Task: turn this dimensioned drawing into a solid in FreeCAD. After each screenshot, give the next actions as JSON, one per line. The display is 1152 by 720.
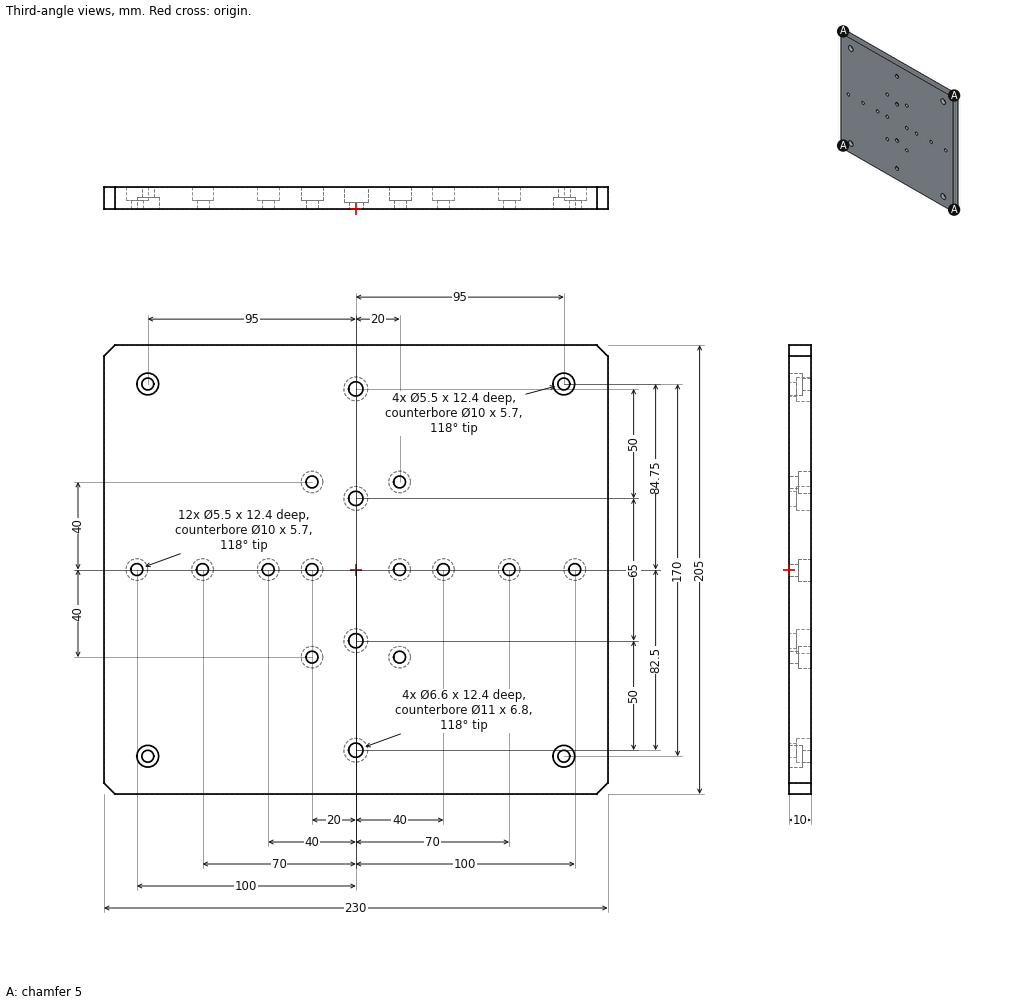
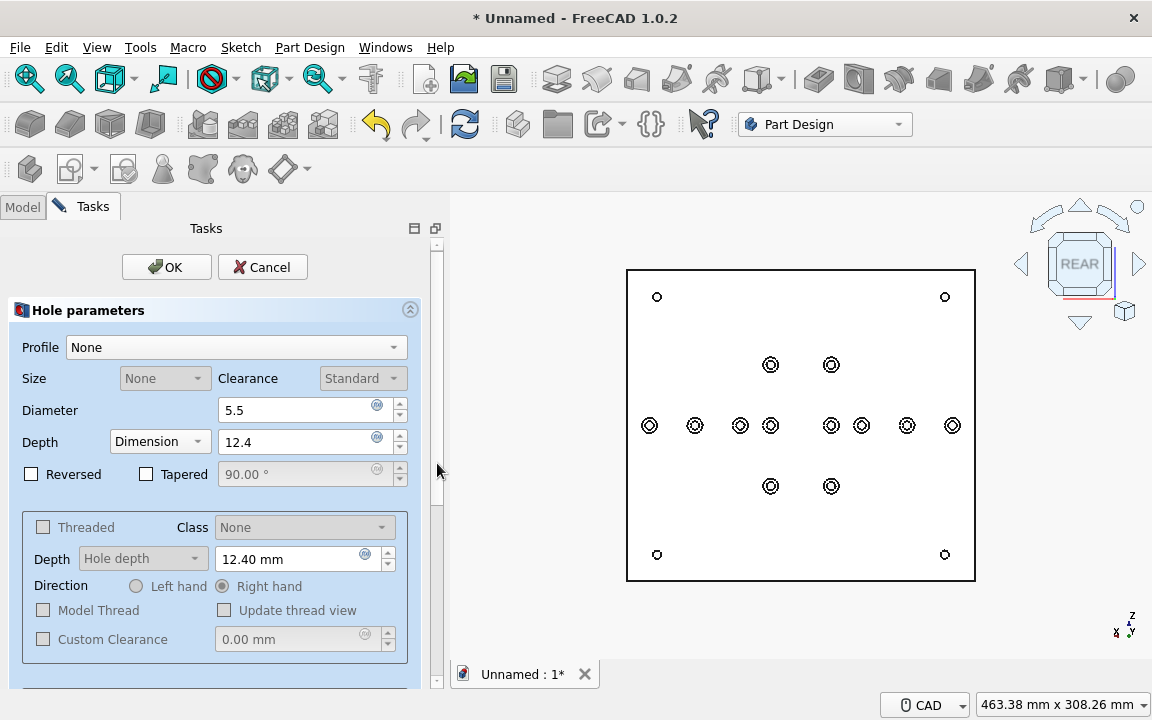
{"action": "left_click", "coordinate": [167, 267]}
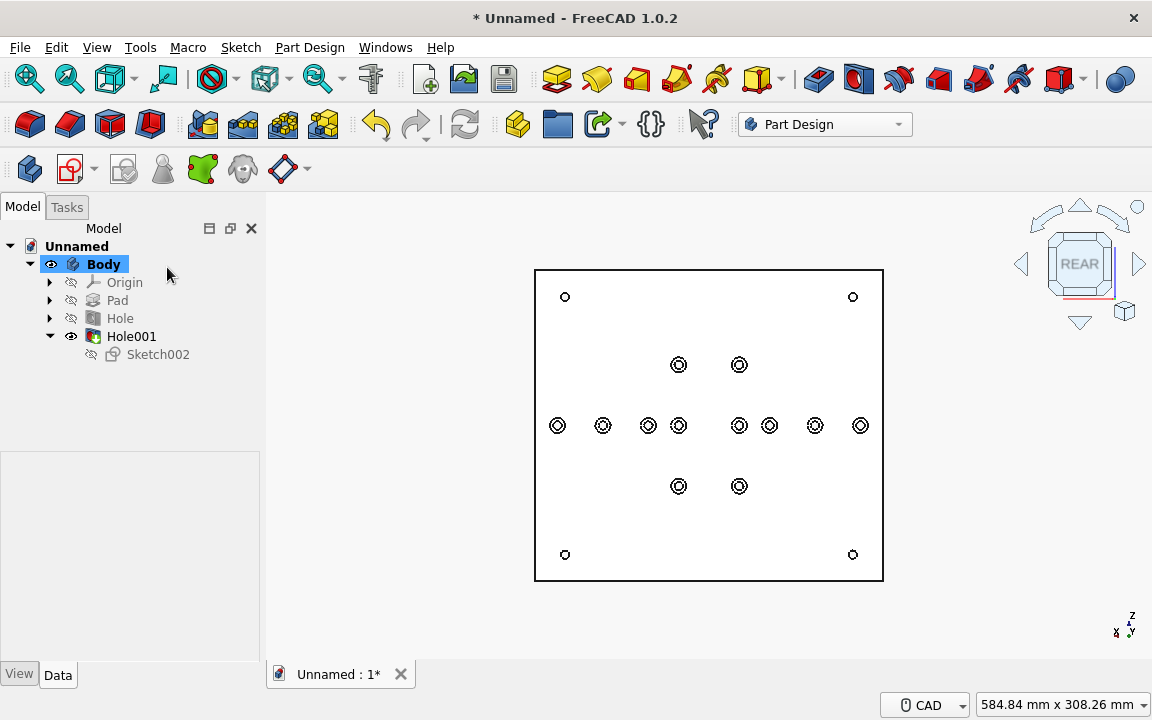
{"action": "scroll", "coordinate": [535, 269], "scroll_direction": "up", "scroll_amount": 5}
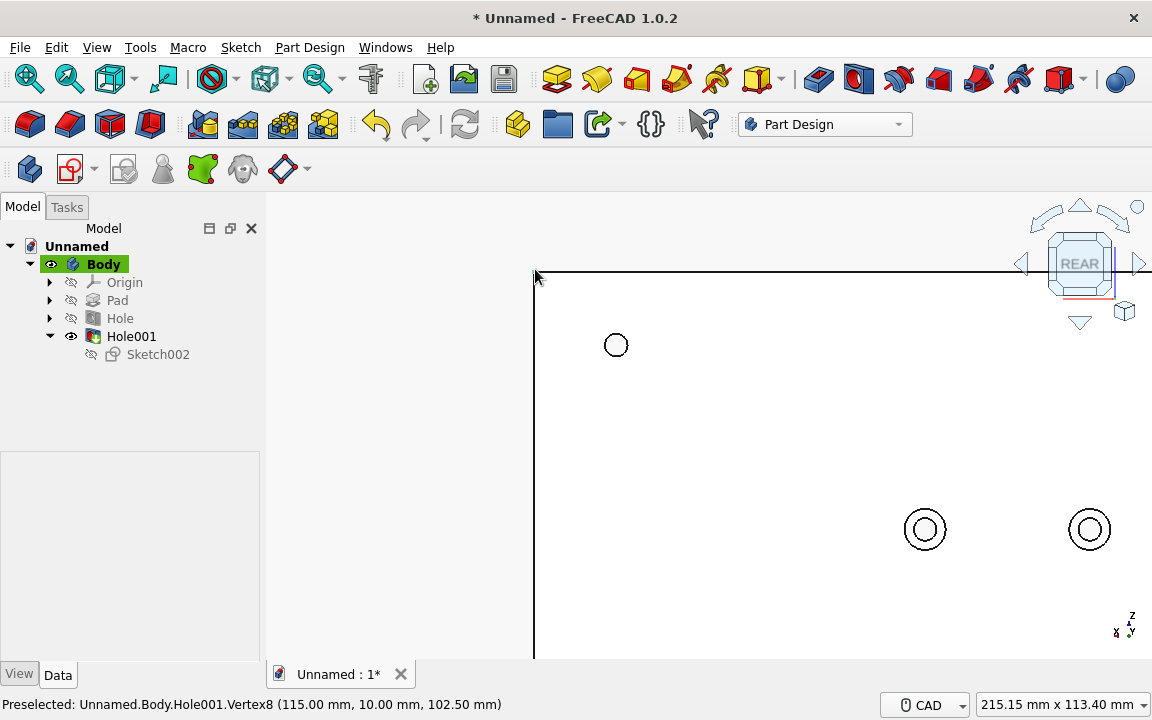
{"action": "left_click", "coordinate": [30, 80]}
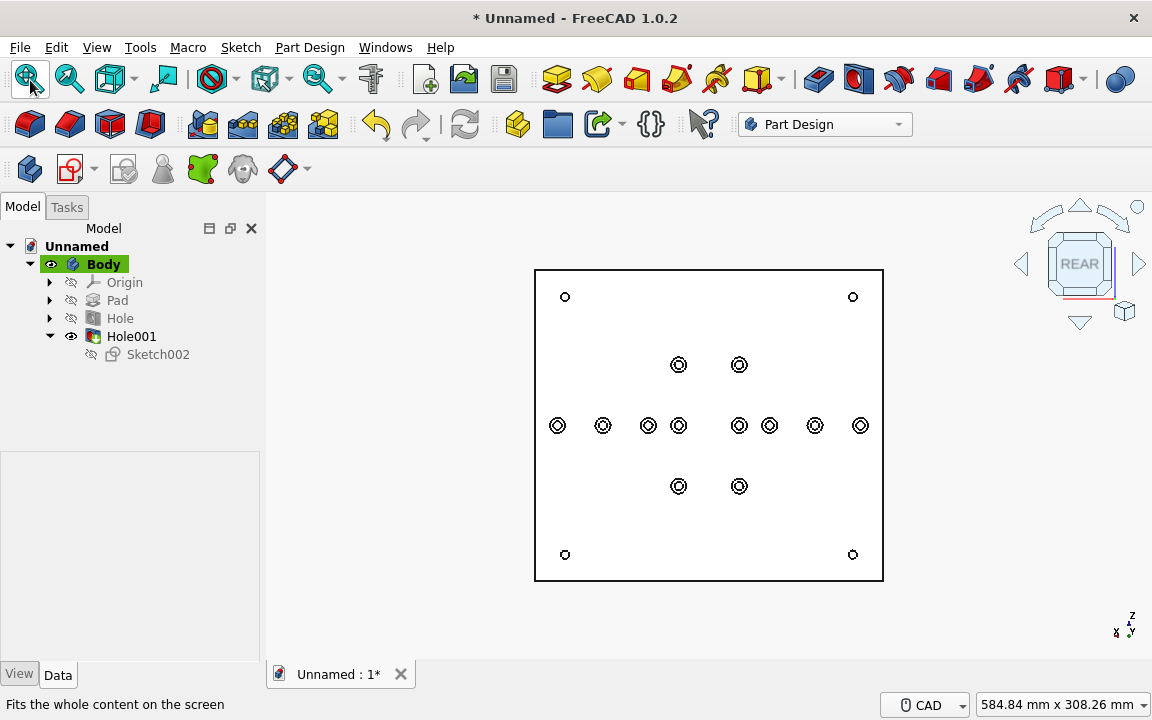
{"action": "key", "text": "0"}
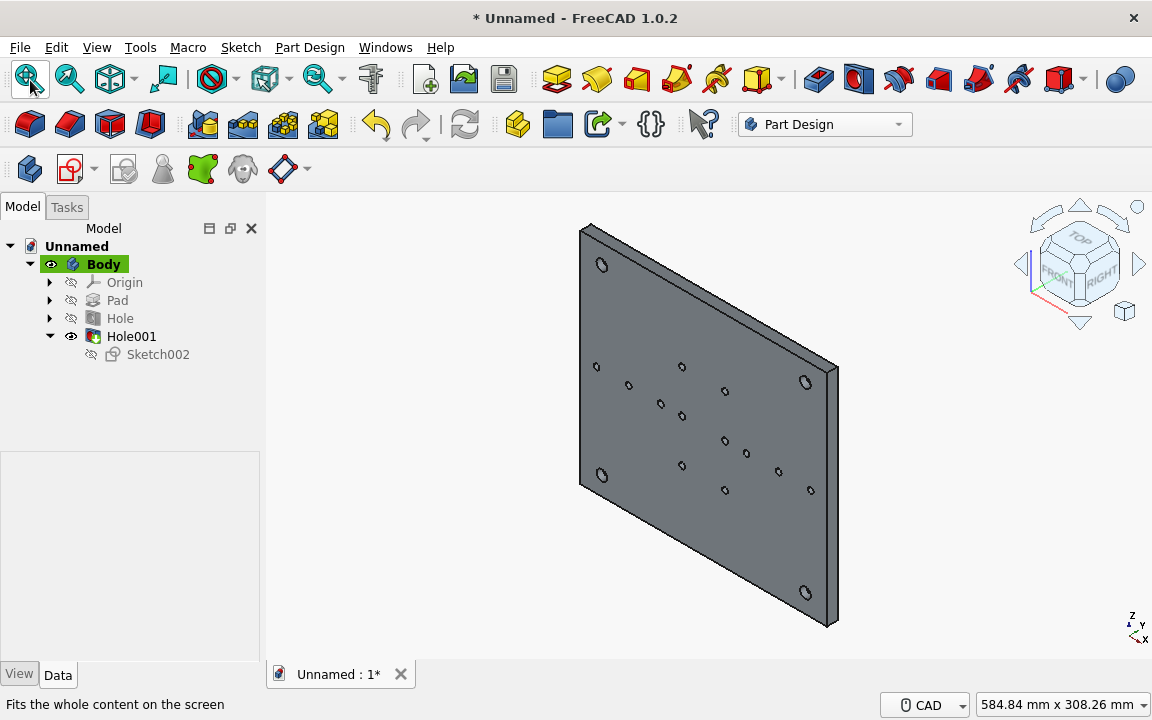
{"action": "left_click", "coordinate": [833, 368]}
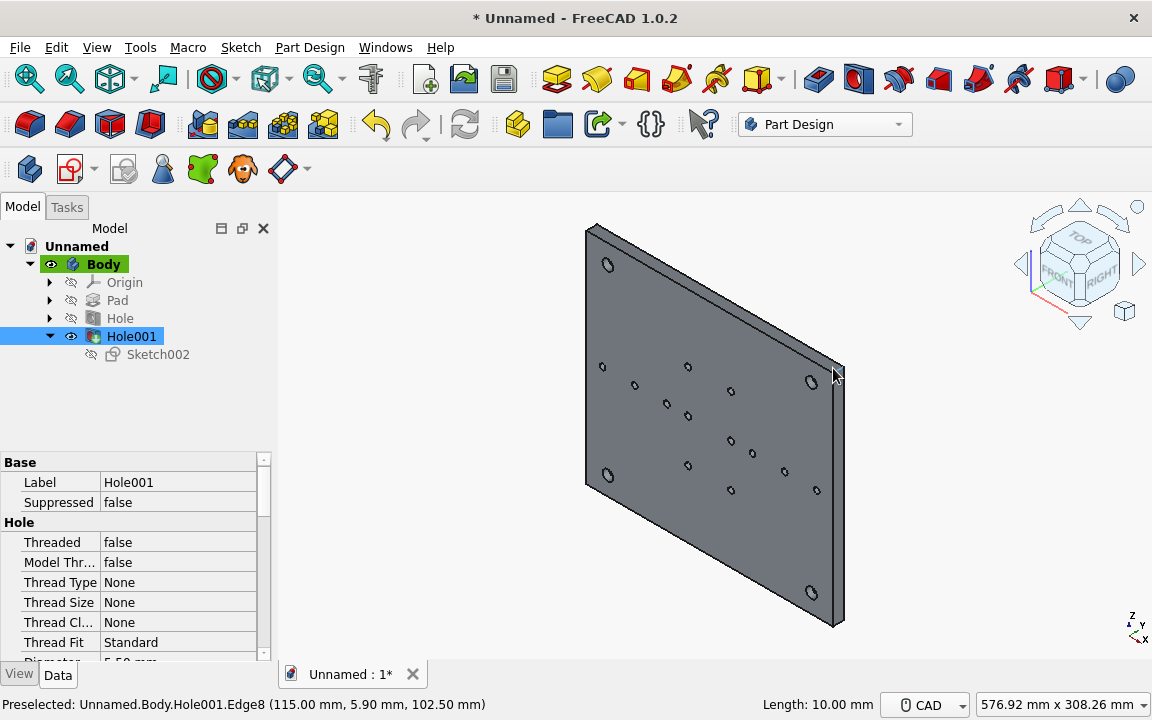
{"action": "scroll", "coordinate": [592, 227], "scroll_direction": "up", "scroll_amount": 5}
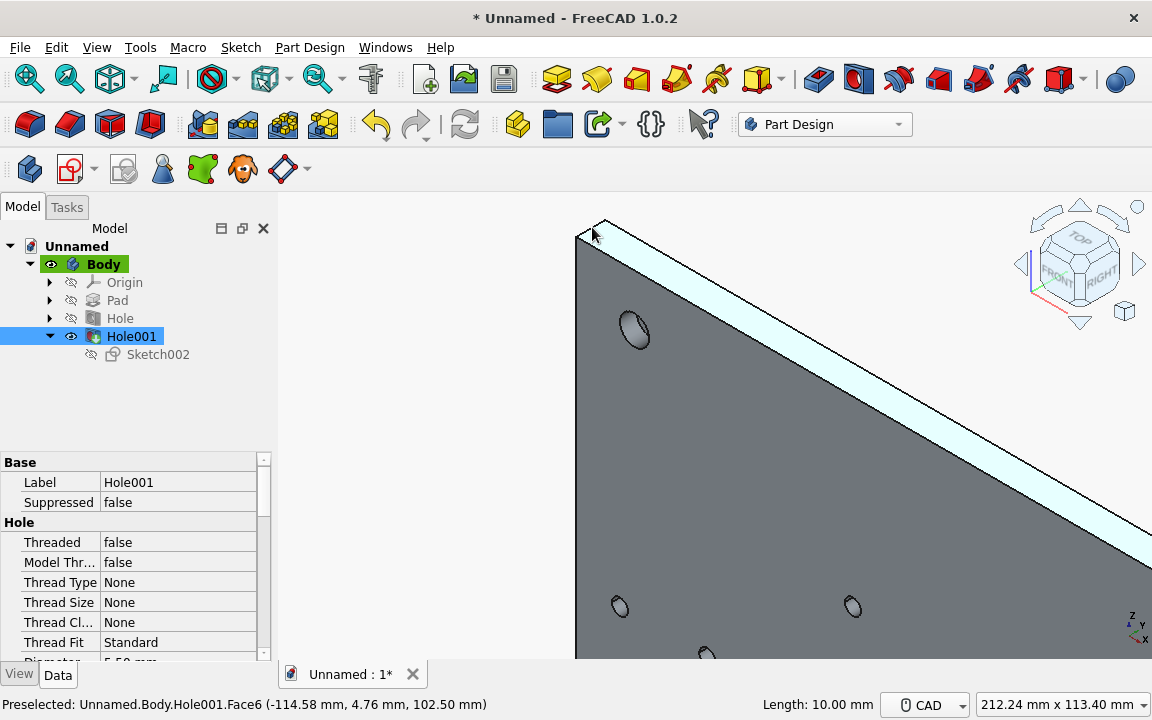
{"action": "left_click", "coordinate": [30, 80]}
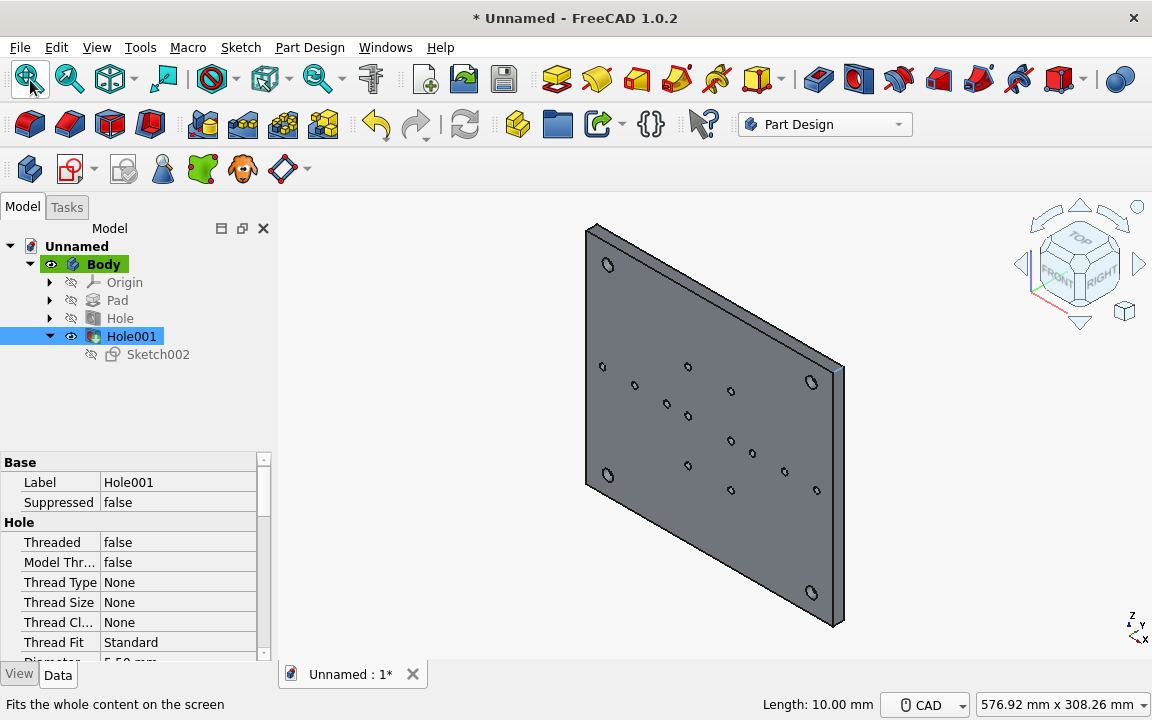
{"action": "key", "text": "2"}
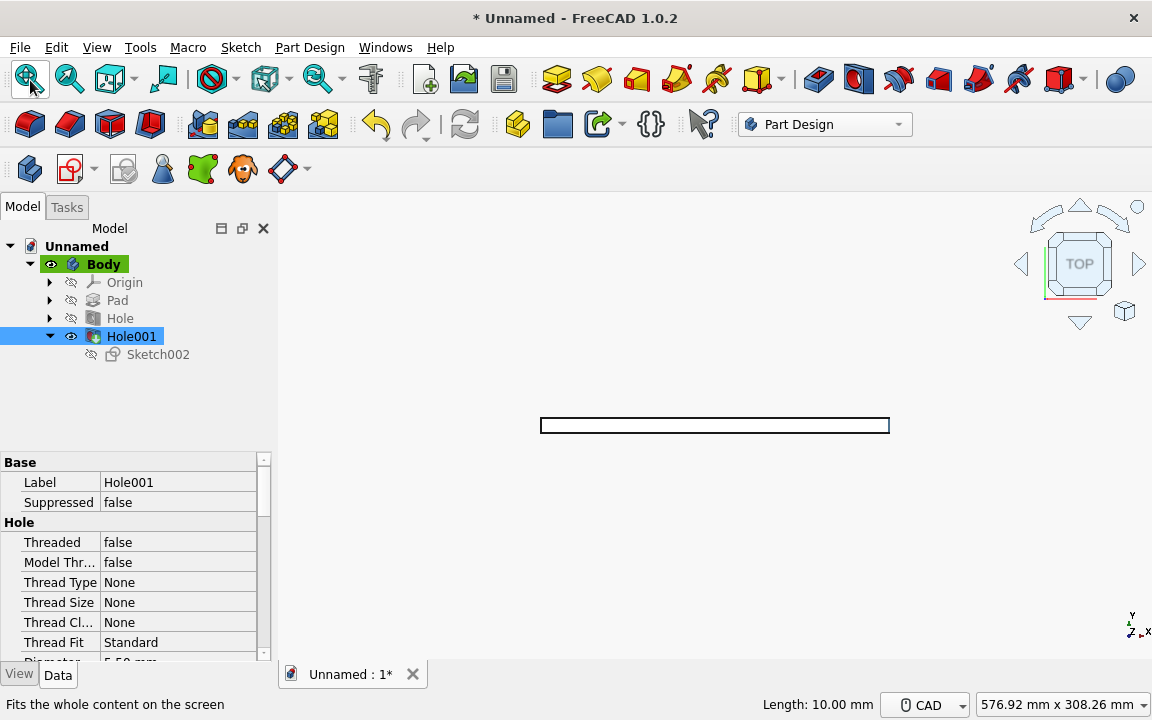
{"action": "left_click", "coordinate": [30, 80]}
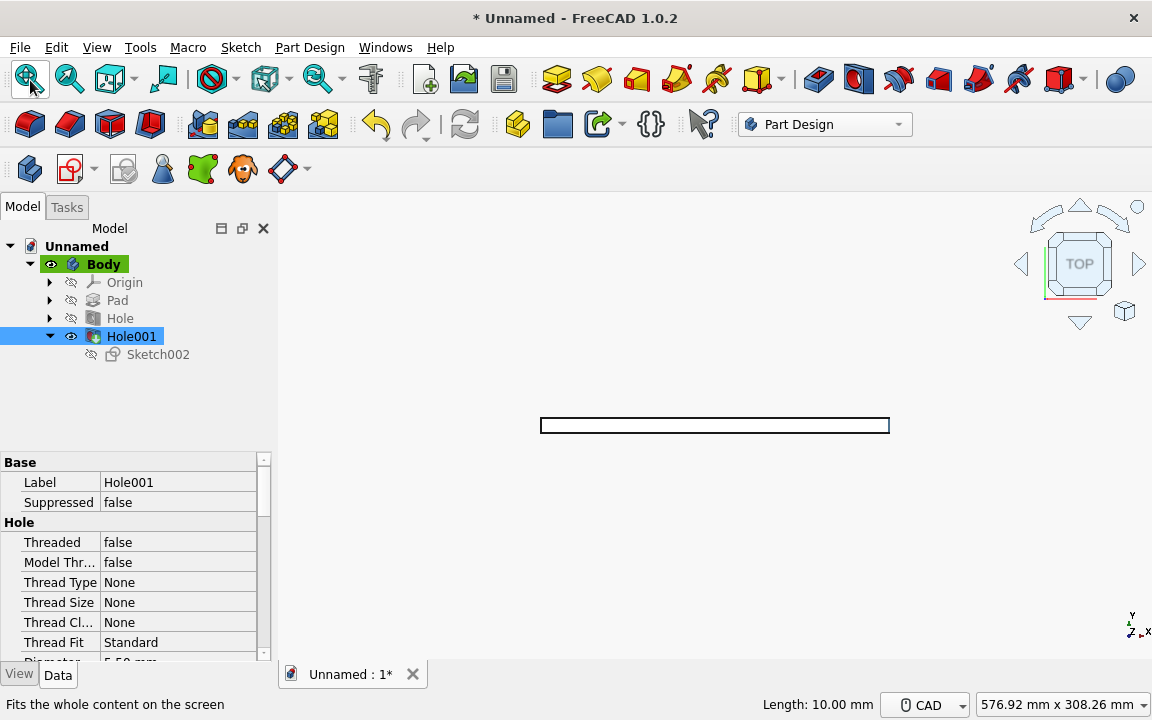
{"action": "left_click", "coordinate": [541, 424], "text": "ctrl"}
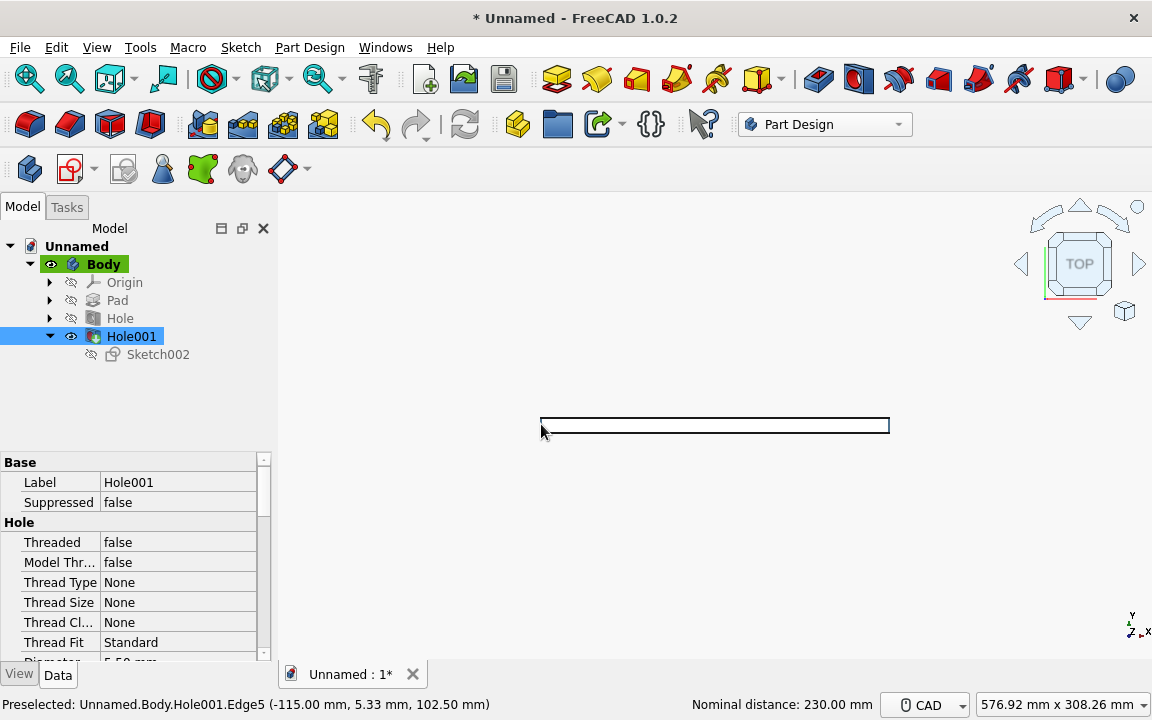
{"action": "scroll", "coordinate": [541, 424], "scroll_direction": "up", "scroll_amount": 5}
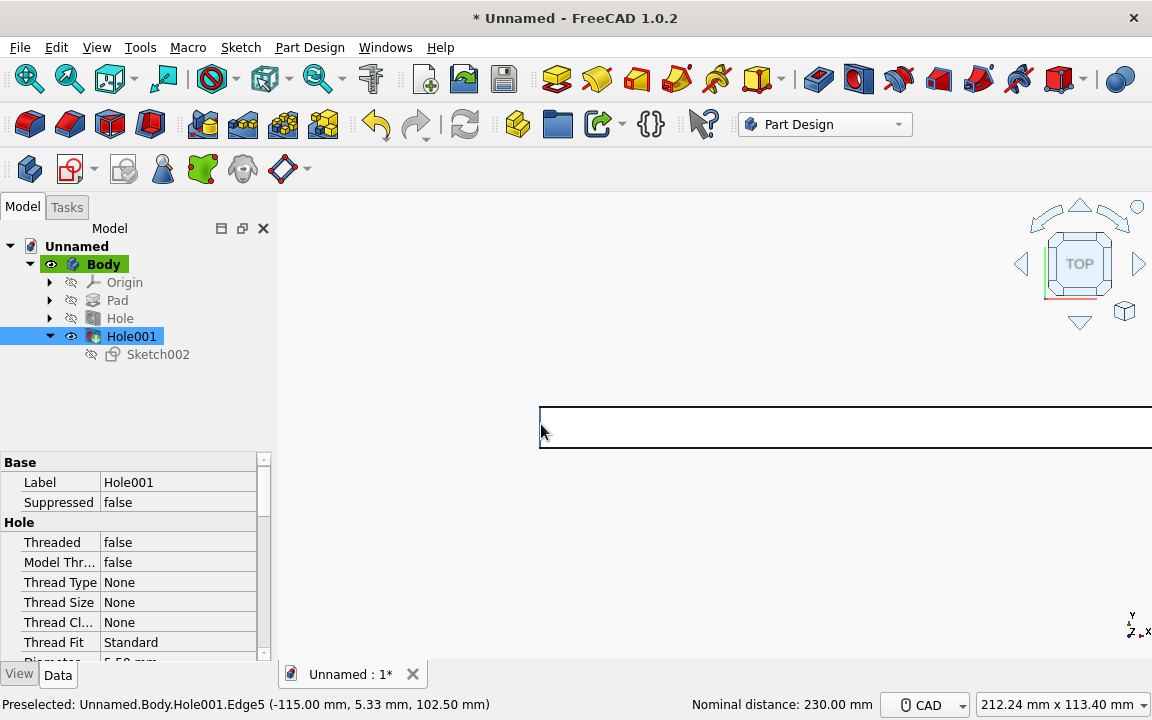
{"action": "left_click", "coordinate": [30, 80]}